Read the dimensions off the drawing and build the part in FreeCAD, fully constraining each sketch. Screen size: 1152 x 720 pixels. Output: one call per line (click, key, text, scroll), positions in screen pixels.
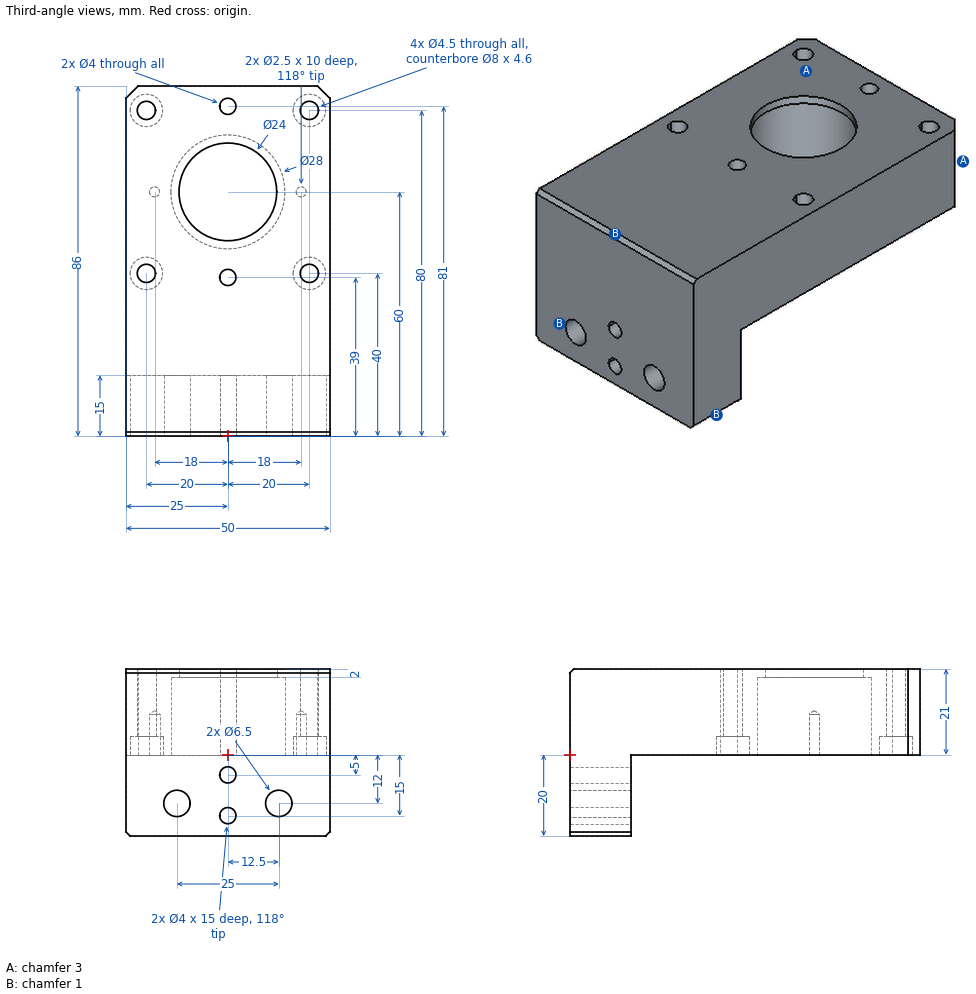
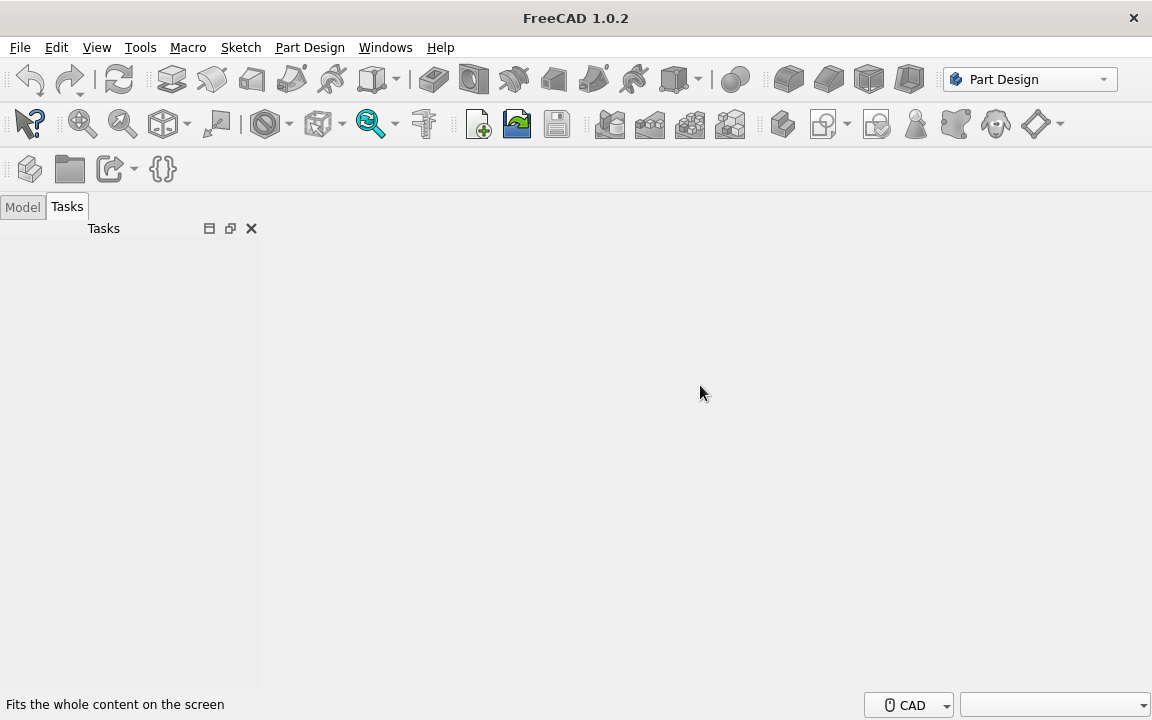
click(478, 124)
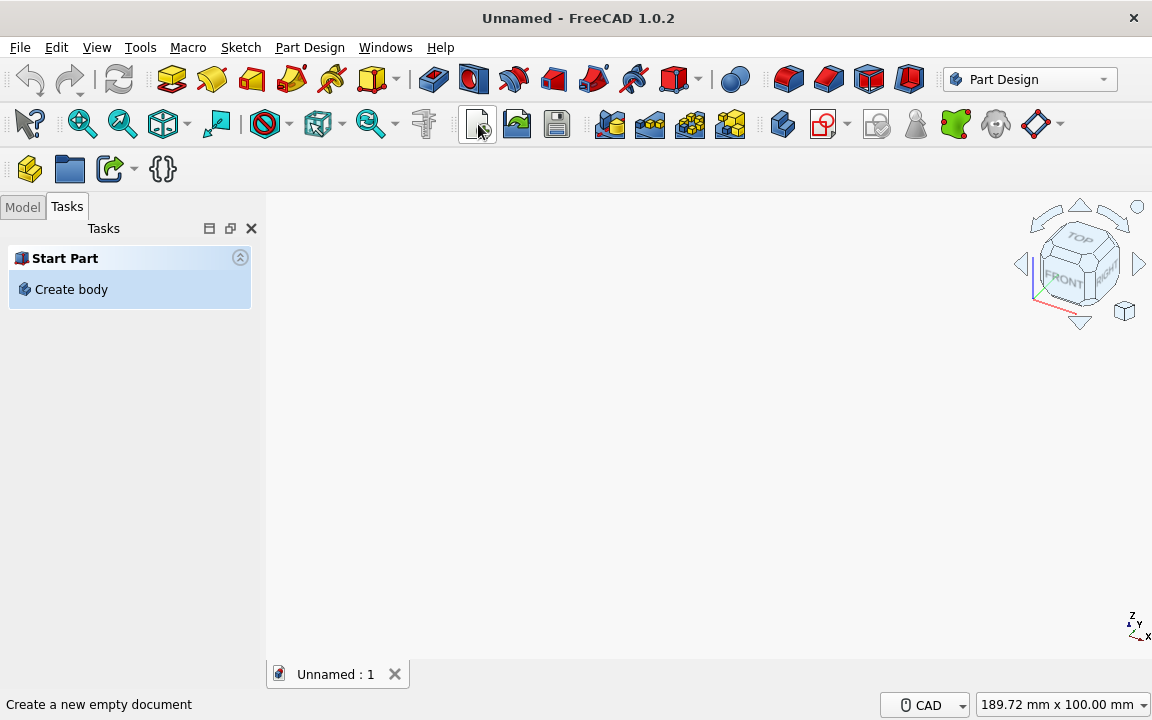
click(824, 124)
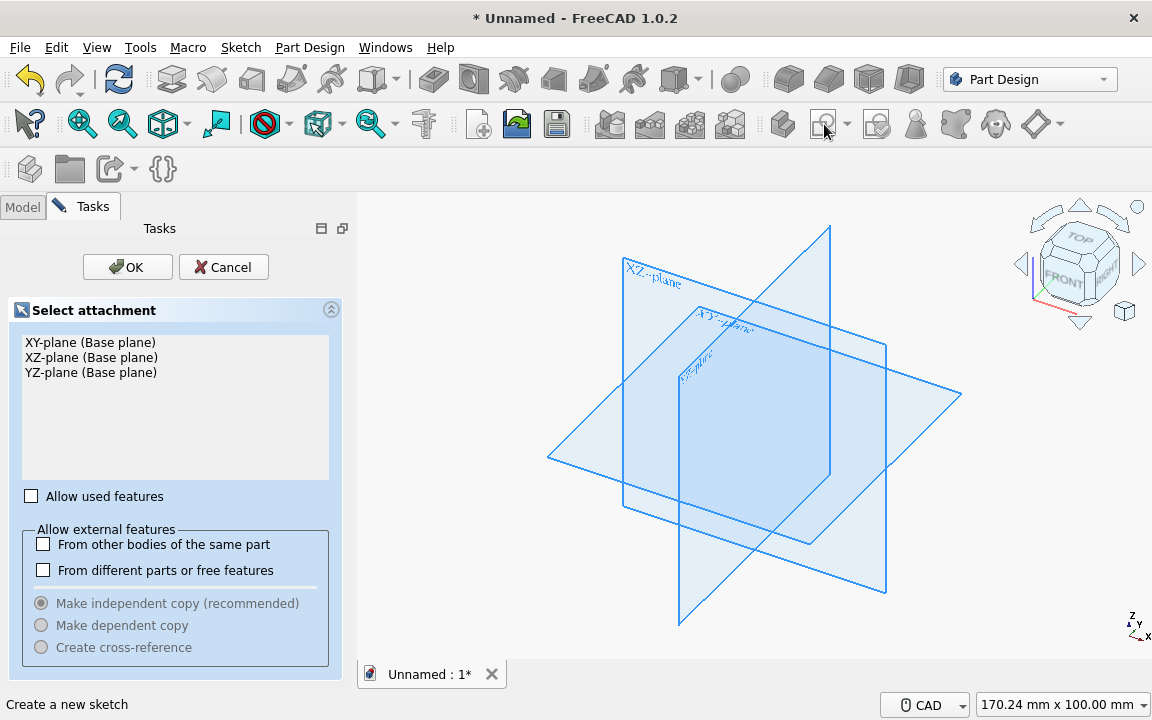
click(82, 342)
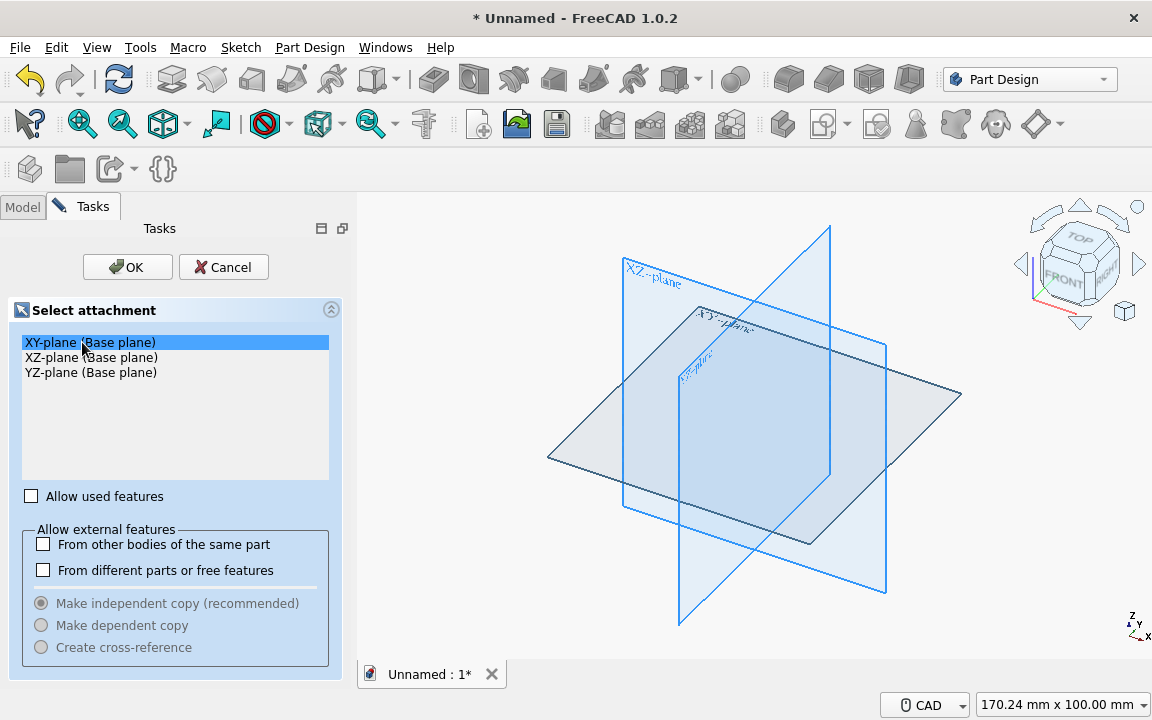
click(128, 267)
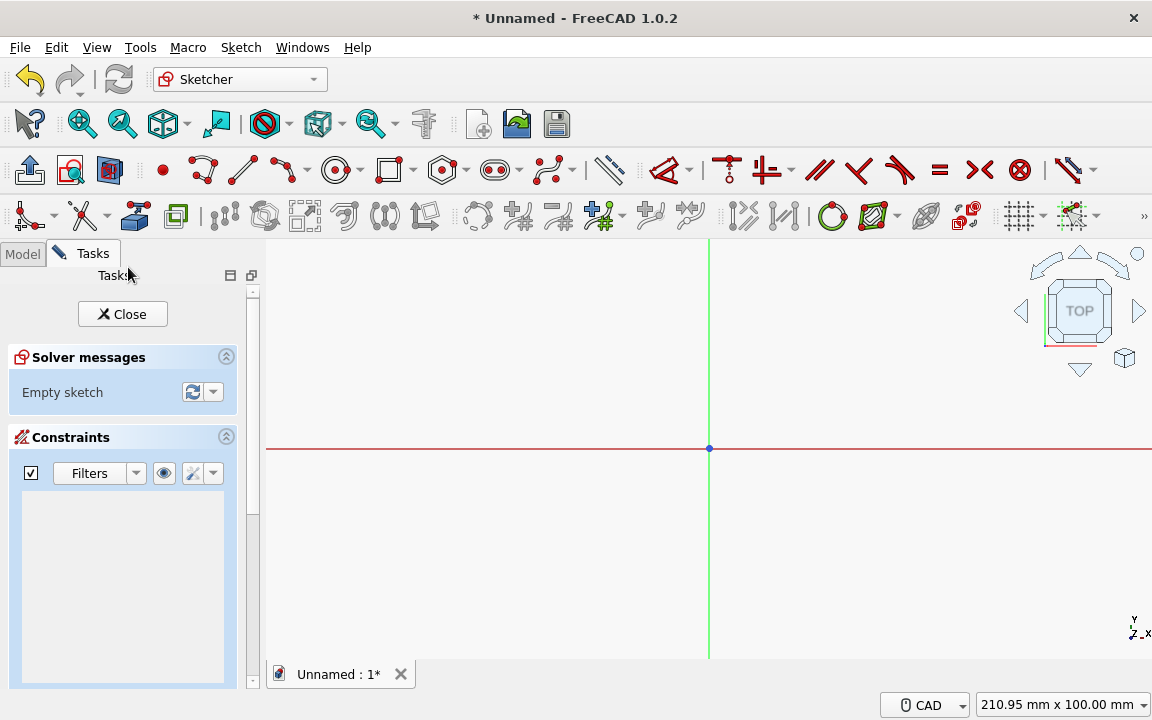
scroll(557, 631, down, 3)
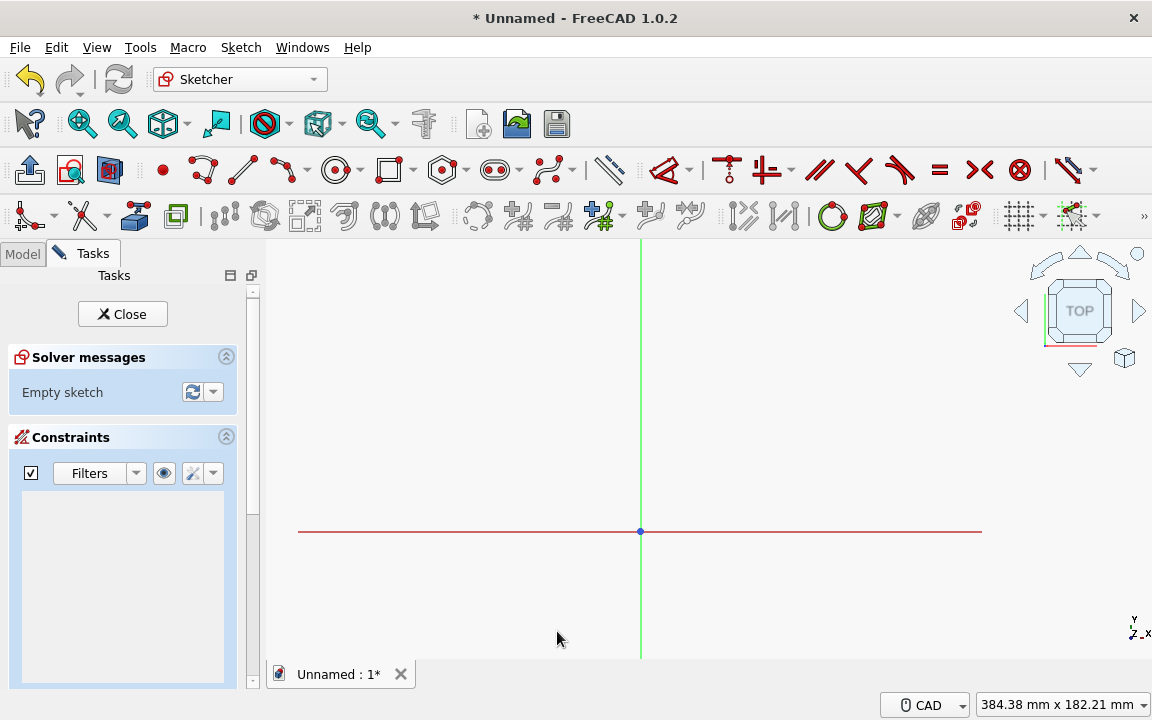
click(390, 170)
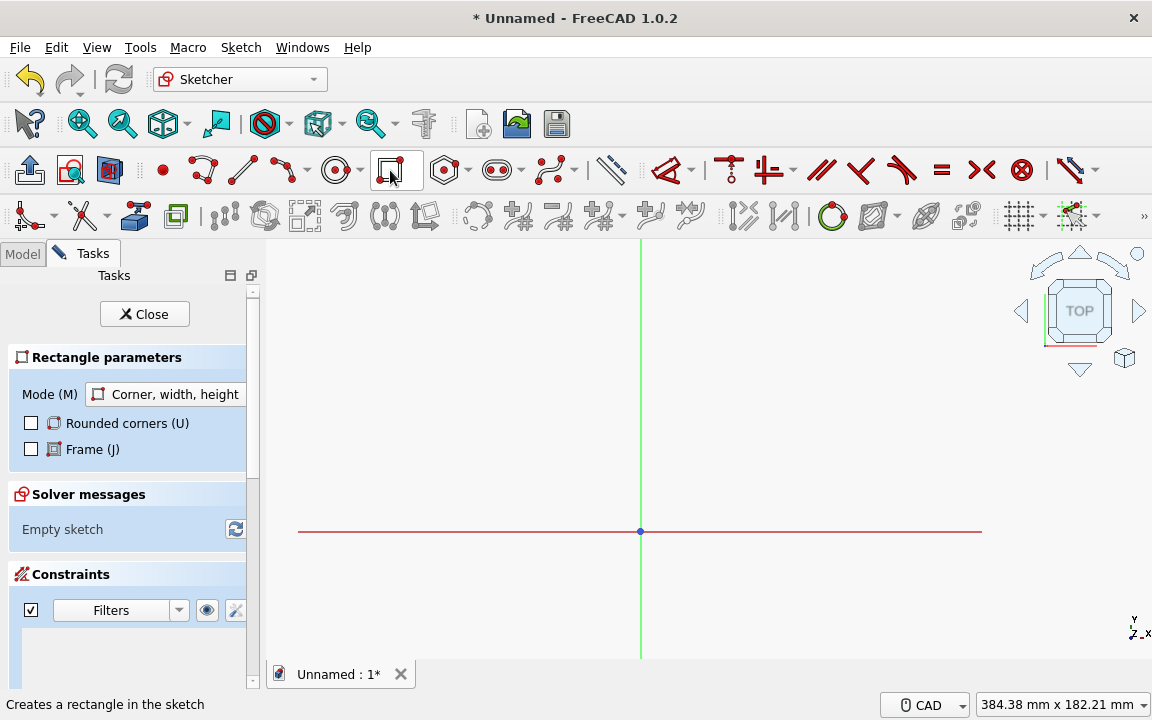
click(583, 333)
click(698, 532)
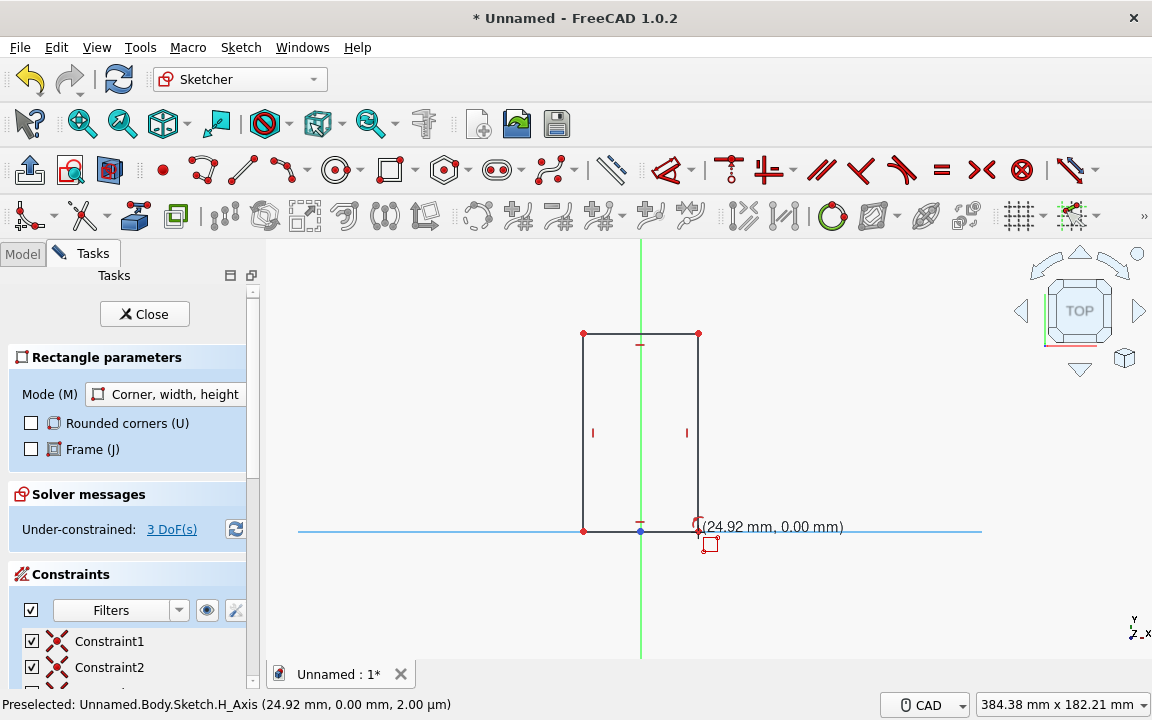
click(336, 170)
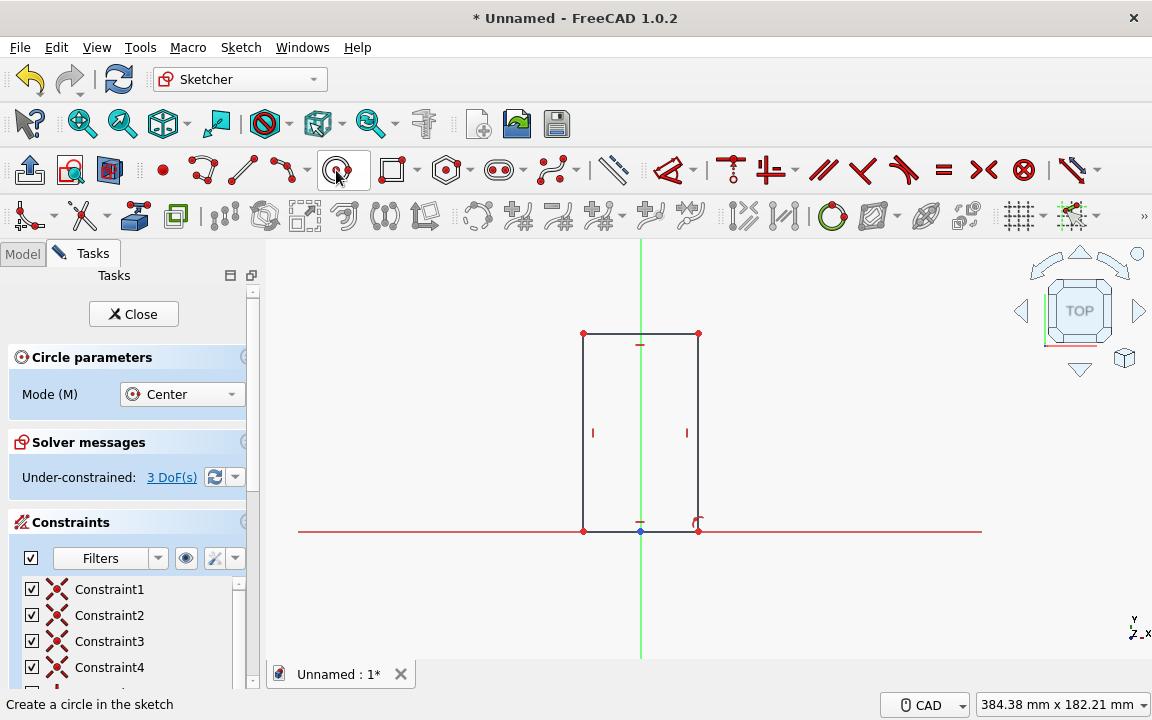
click(641, 393)
click(663, 370)
key(Escape)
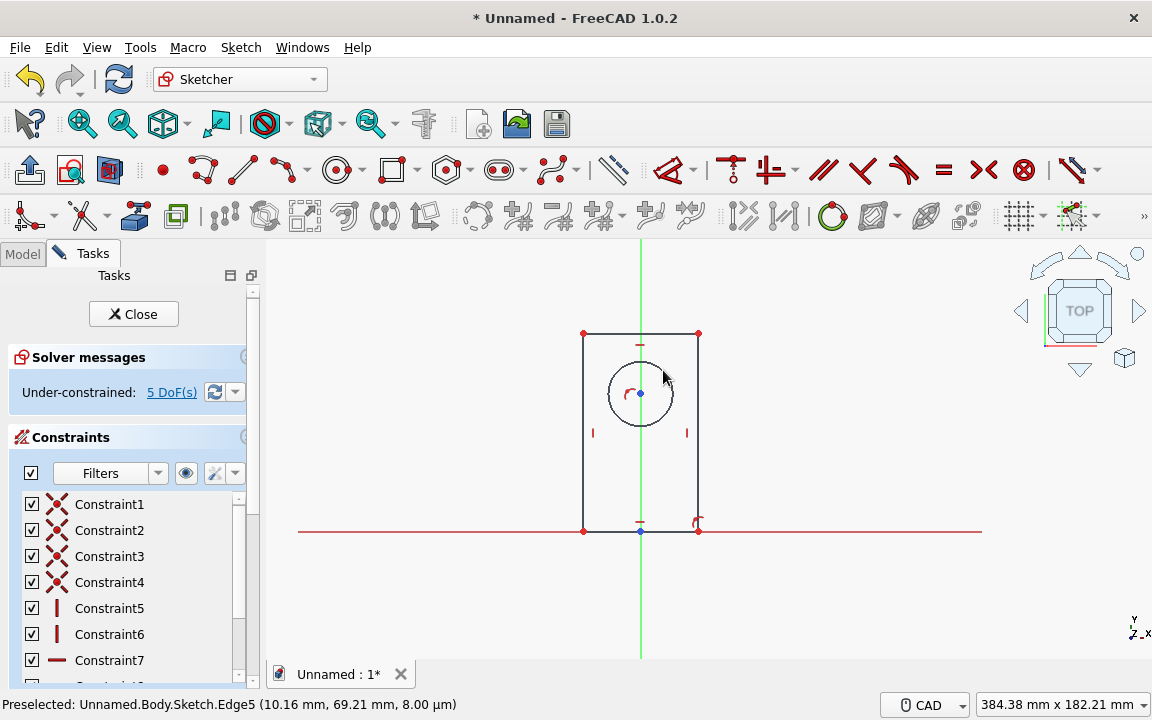
click(663, 371)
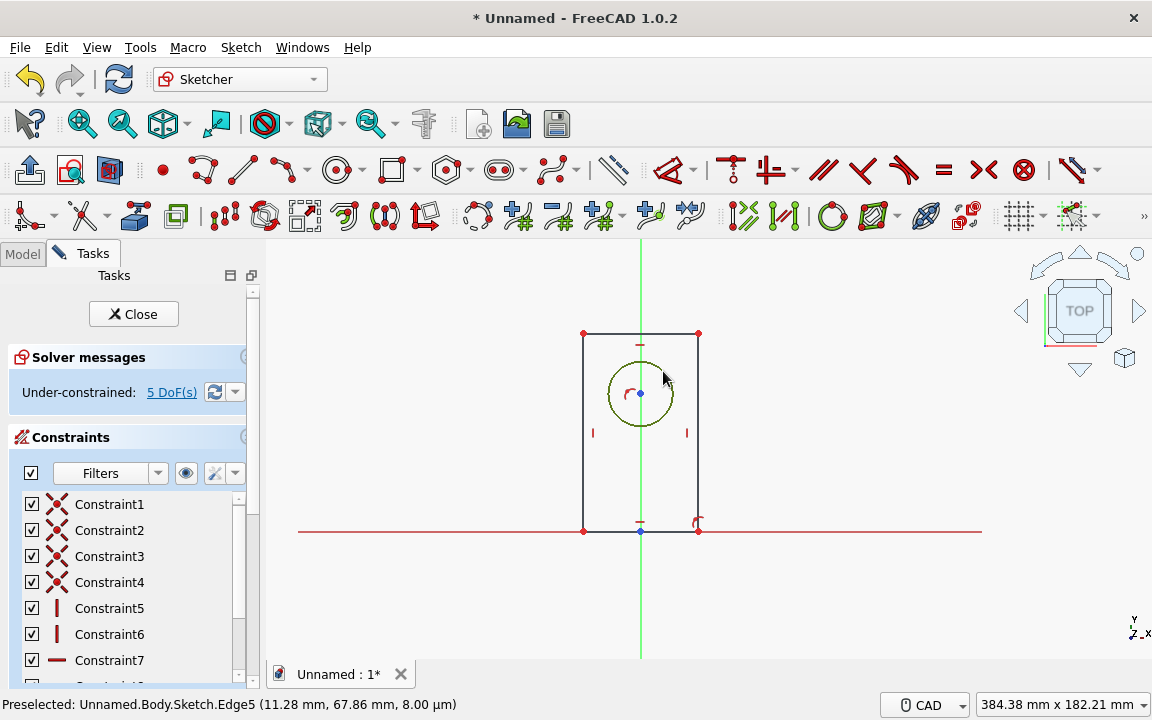
key(k)
key(o)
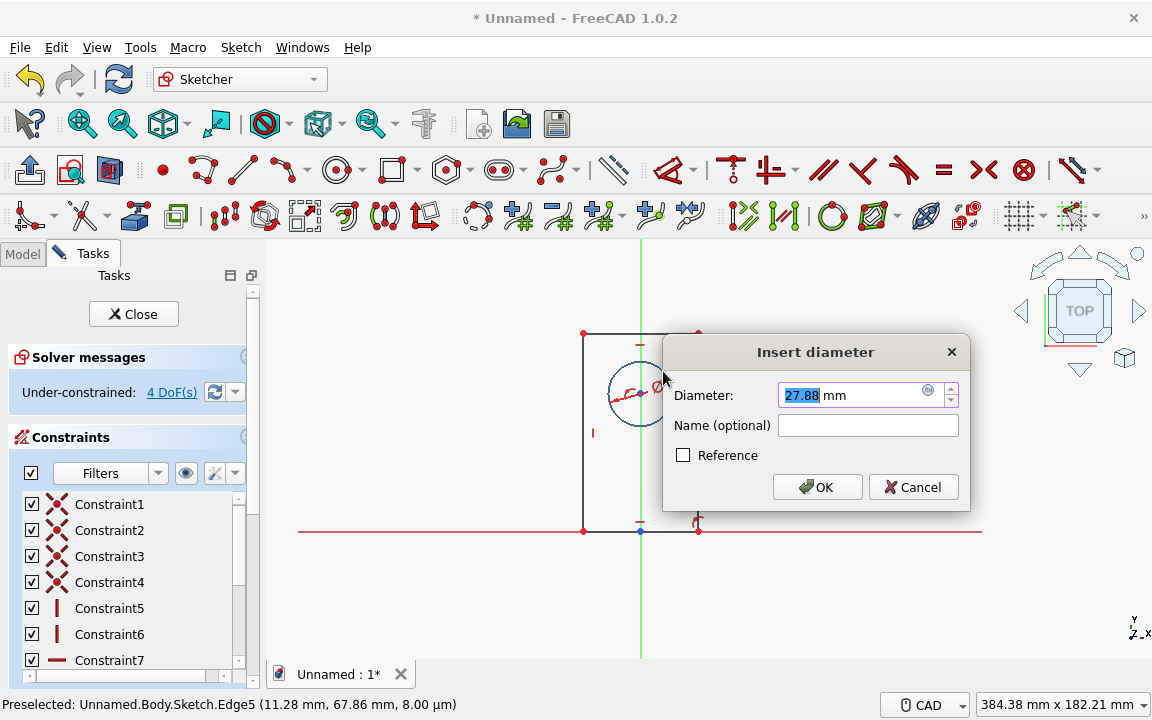
text(28)
key(Return)